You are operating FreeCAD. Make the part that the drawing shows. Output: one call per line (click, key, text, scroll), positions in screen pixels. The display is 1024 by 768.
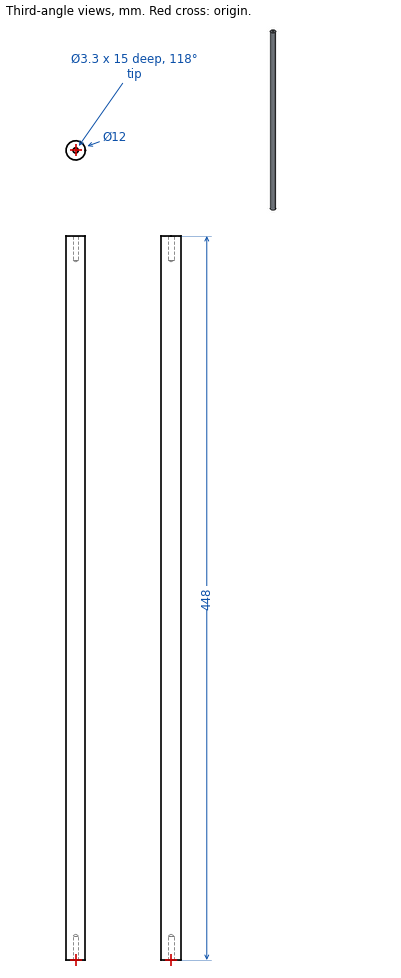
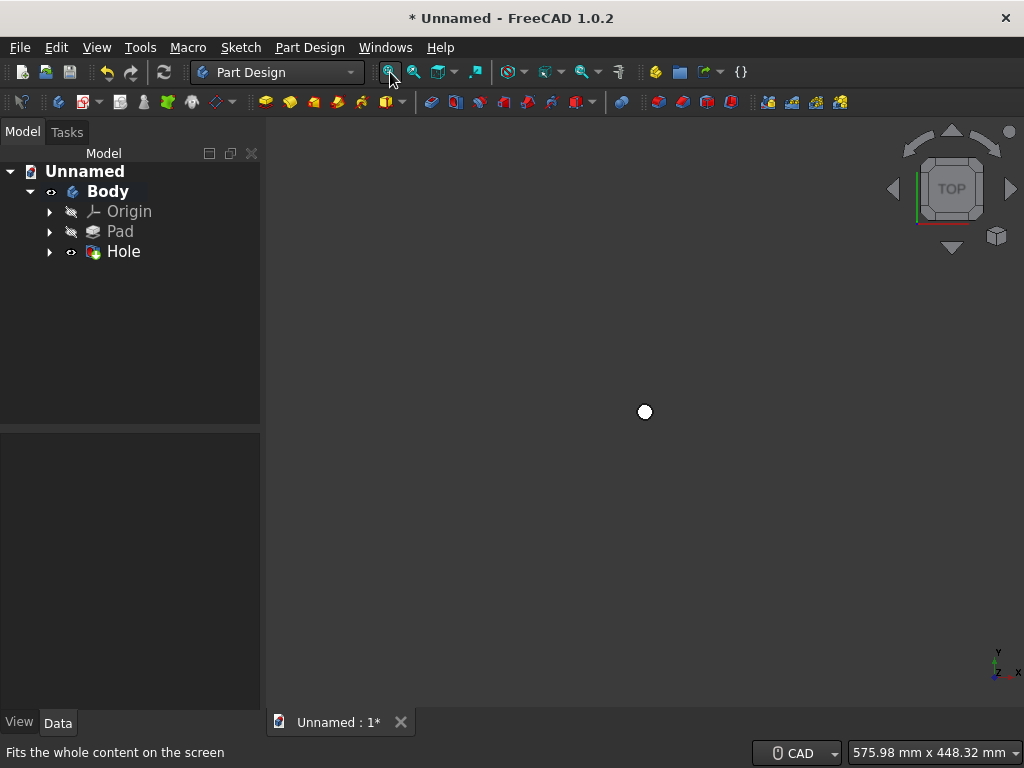
click(390, 72)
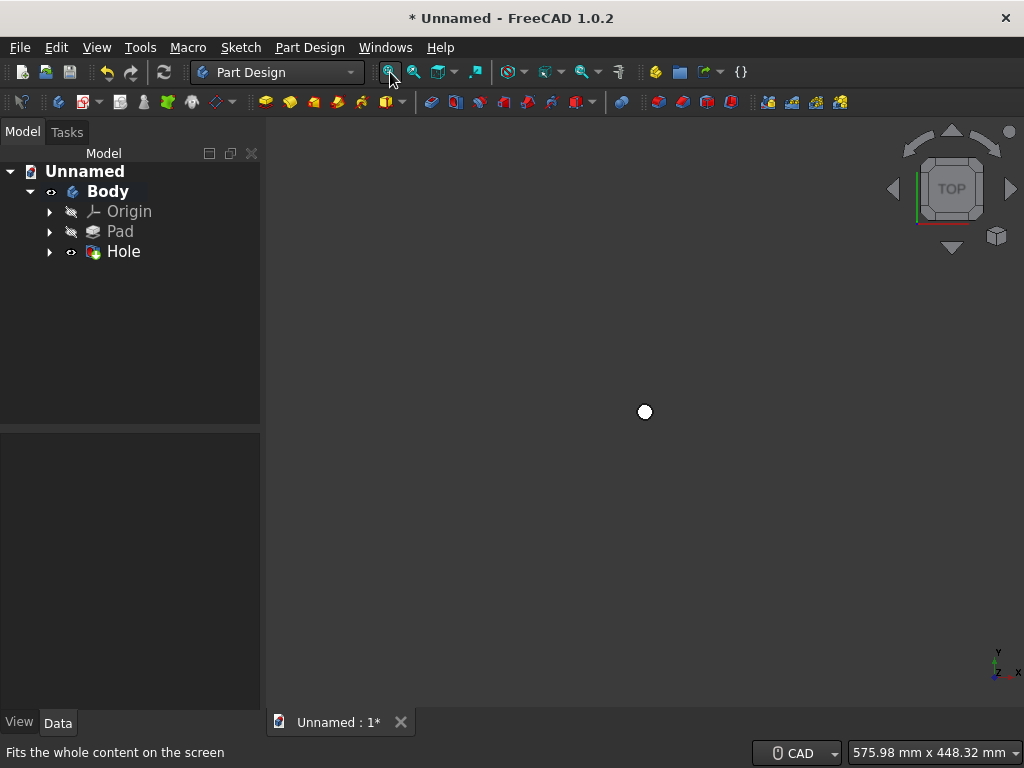
key(1)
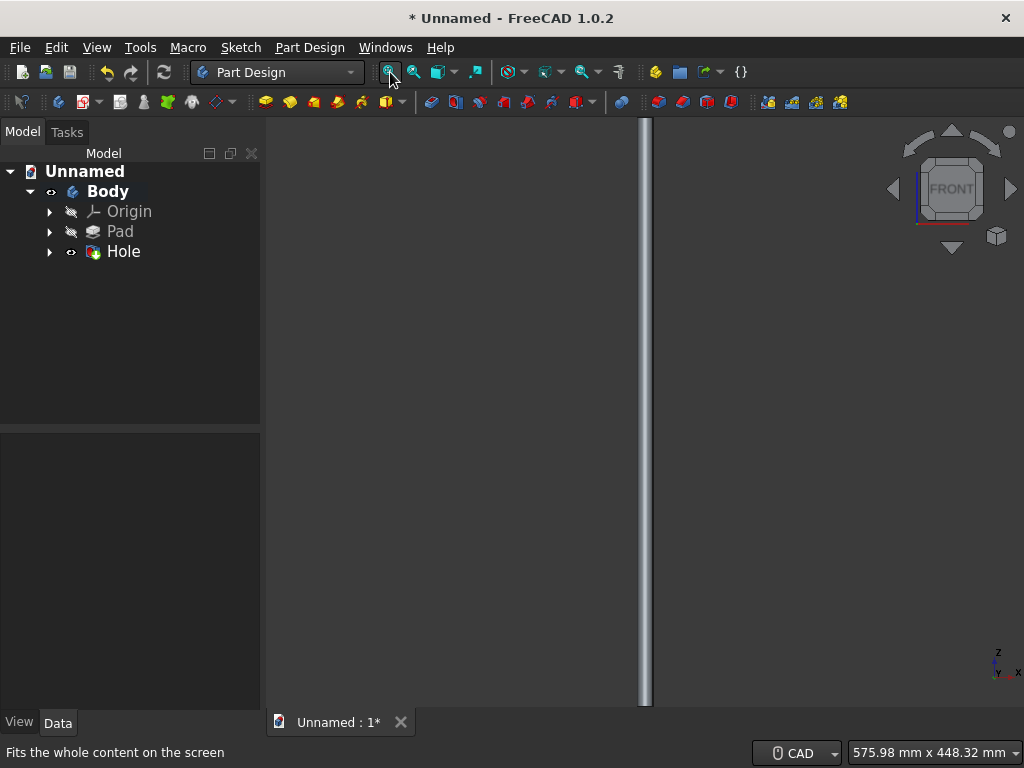
click(390, 72)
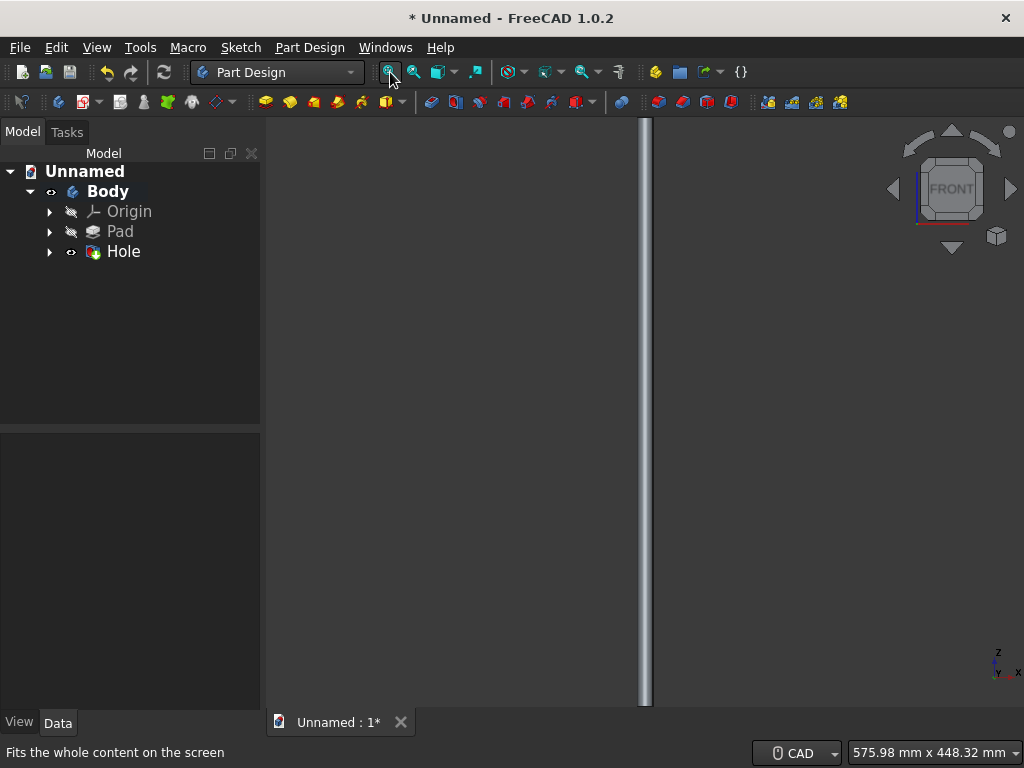
click(50, 212)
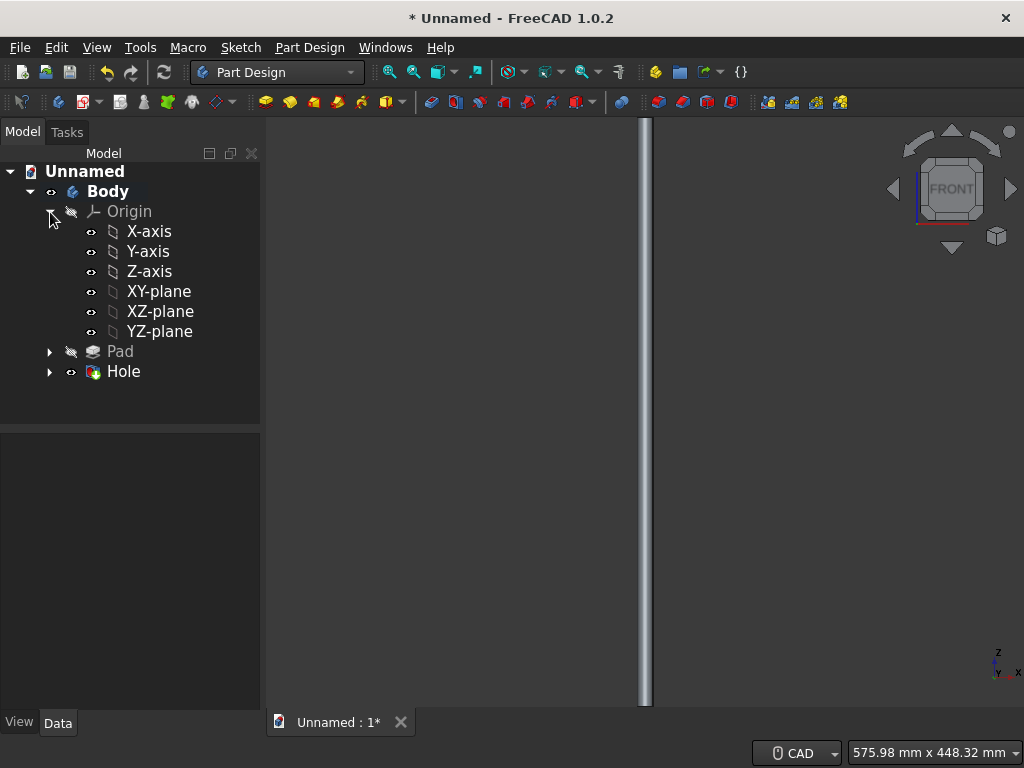
click(136, 292)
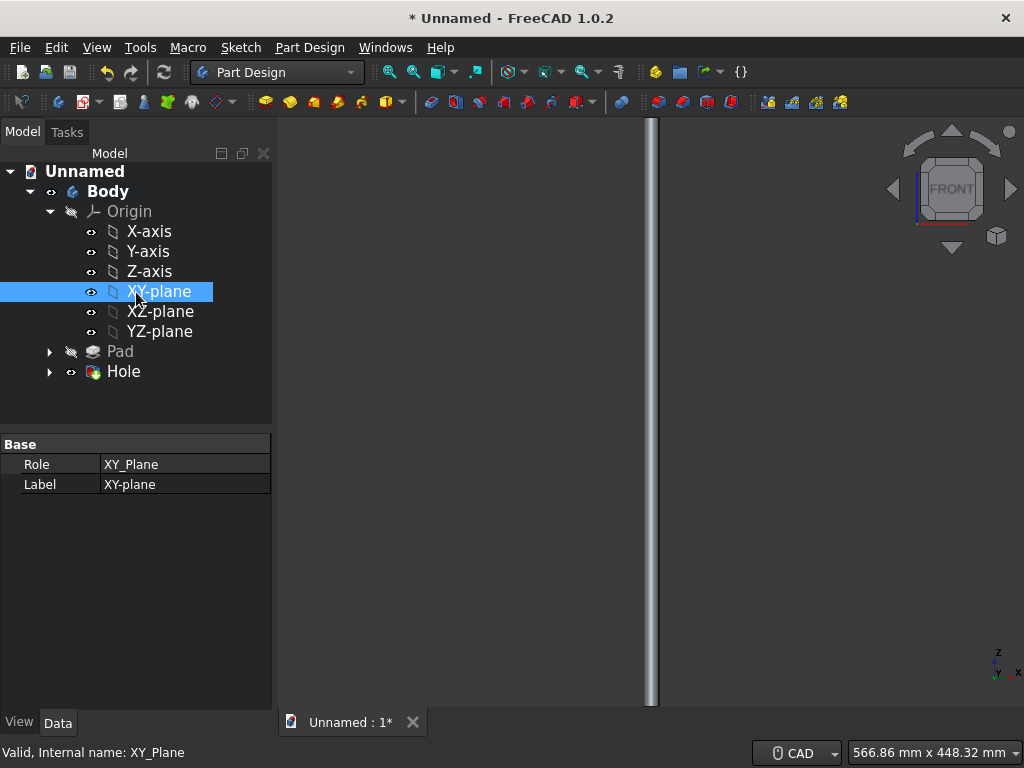
click(216, 102)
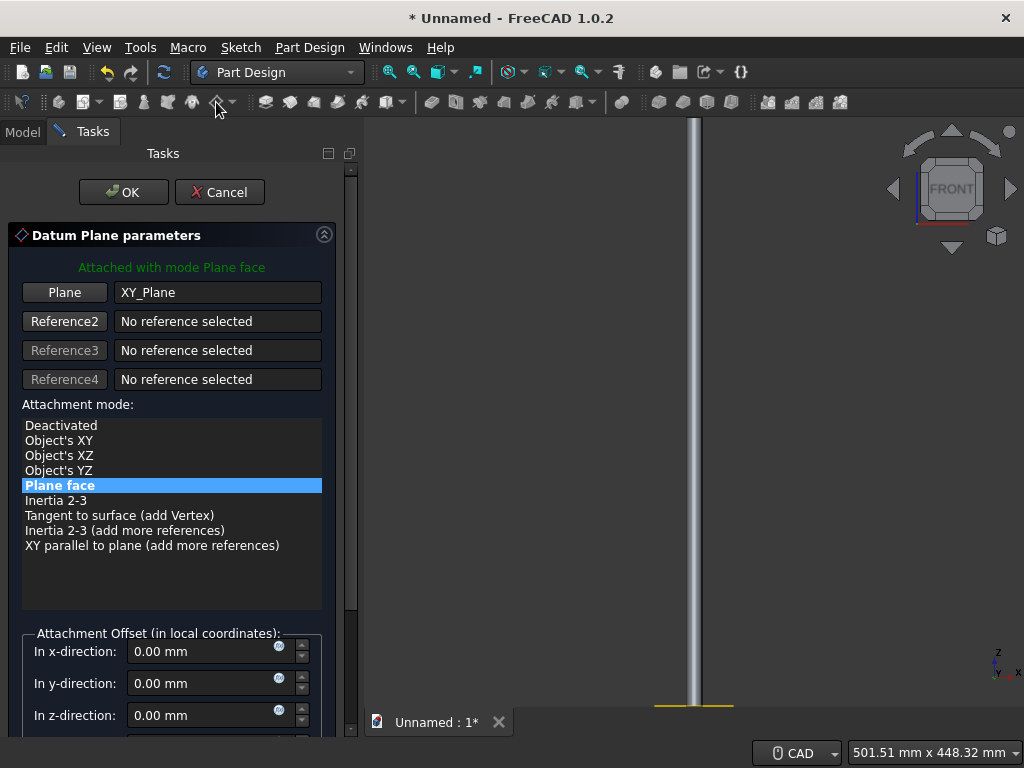
triple_click(210, 715)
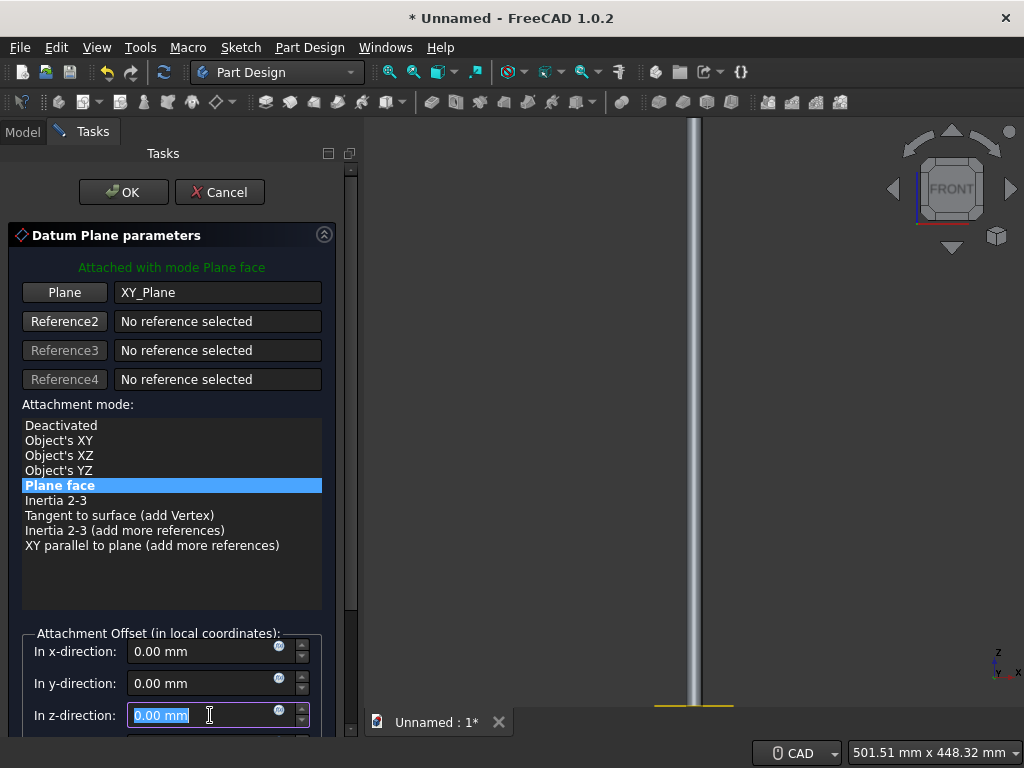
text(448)
key(Tab)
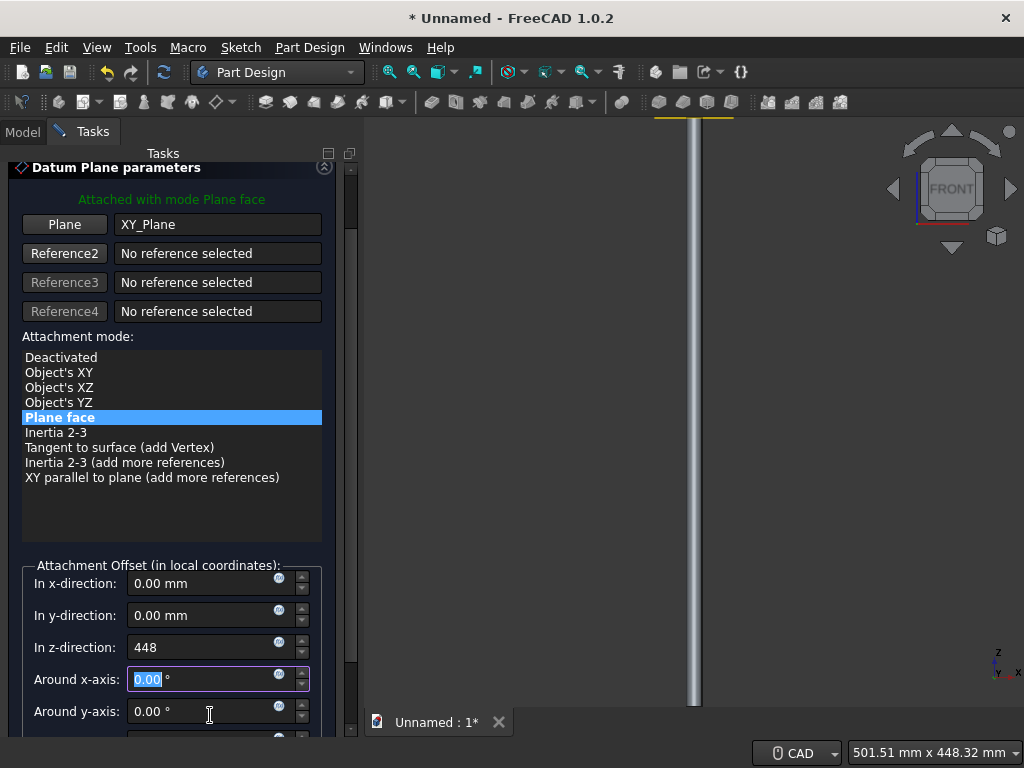
scroll(351, 450, up, 2)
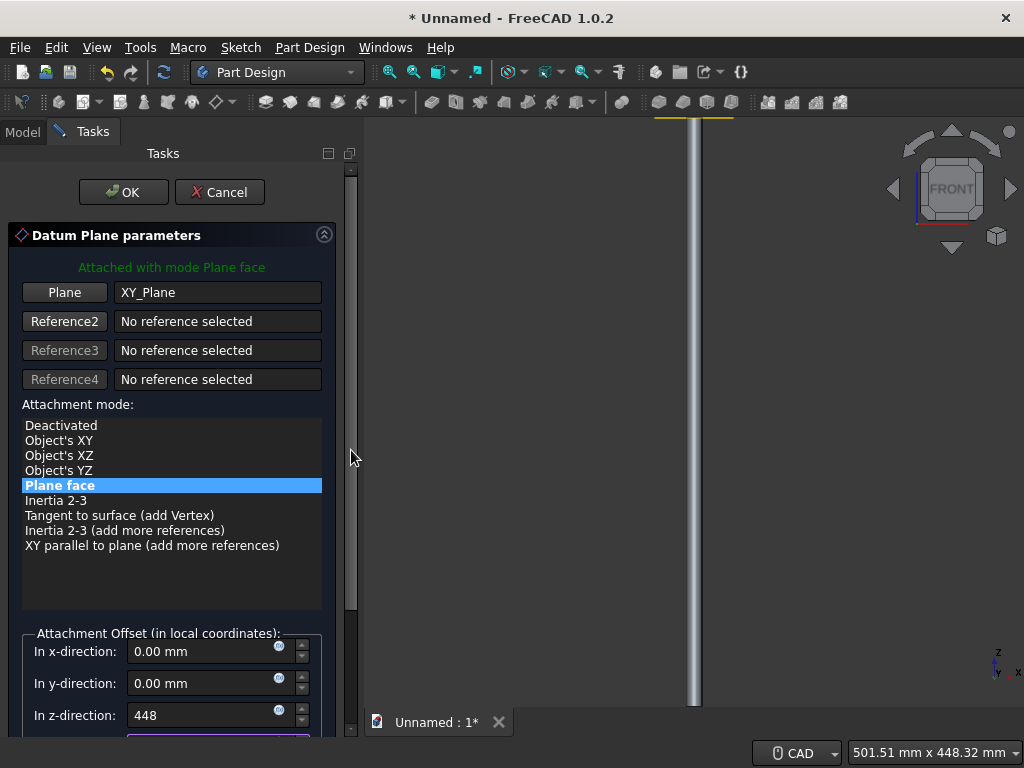
click(124, 192)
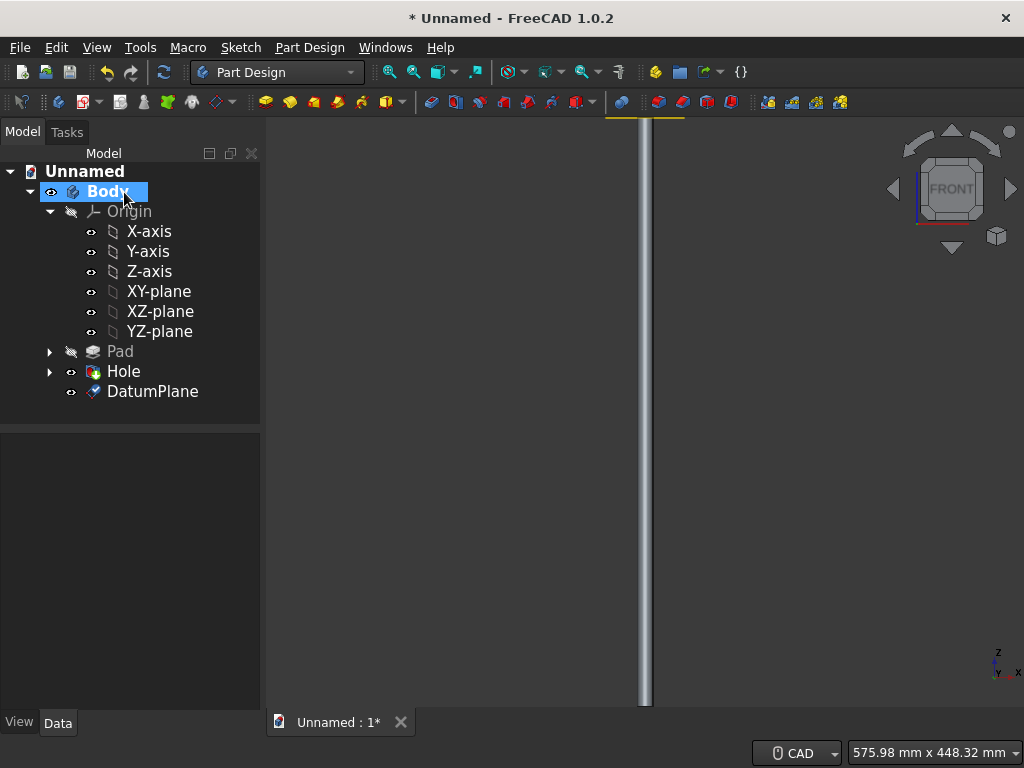
click(116, 392)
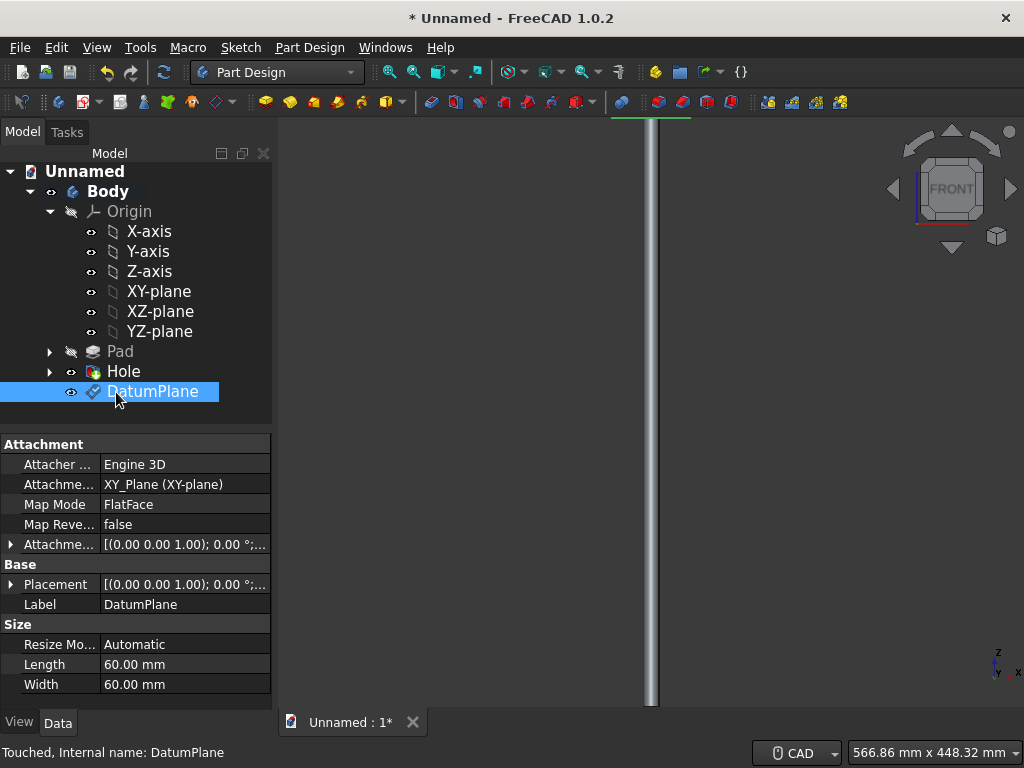
click(84, 102)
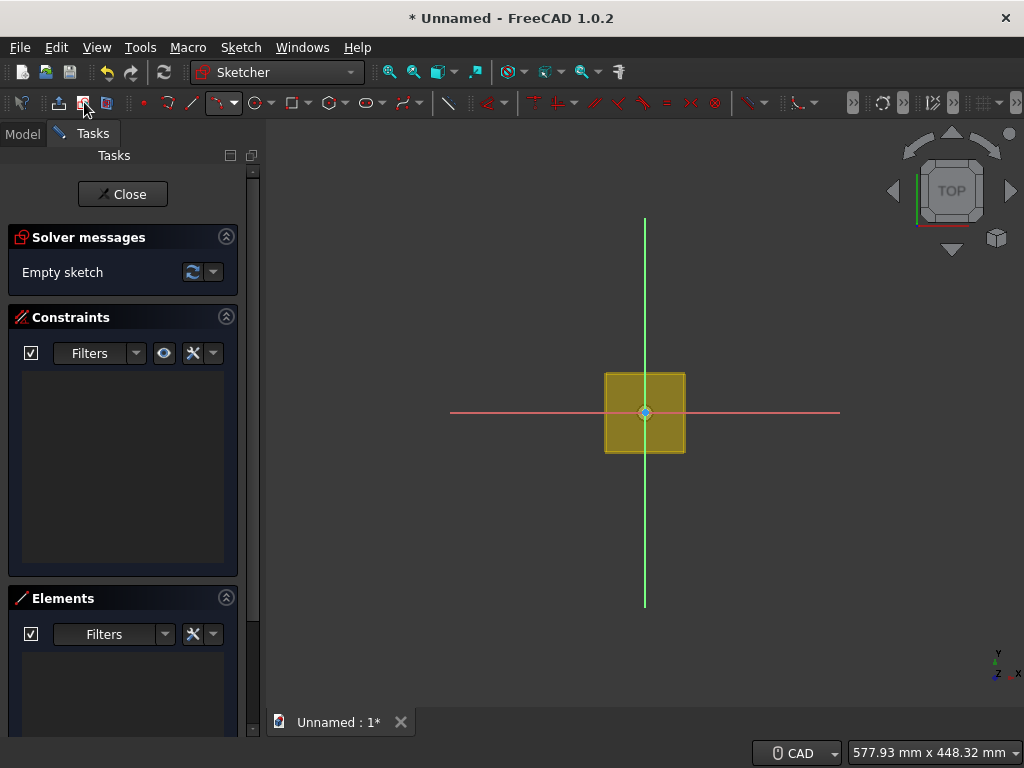
scroll(649, 413, up, 15)